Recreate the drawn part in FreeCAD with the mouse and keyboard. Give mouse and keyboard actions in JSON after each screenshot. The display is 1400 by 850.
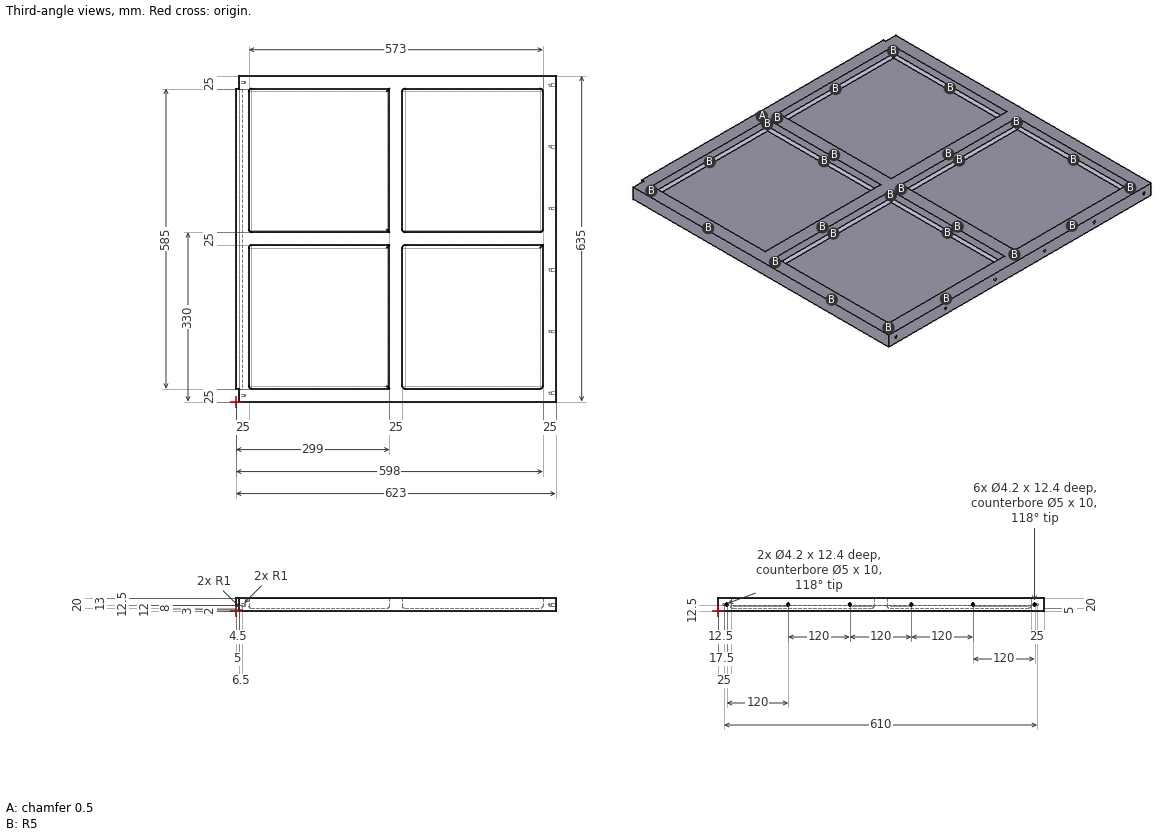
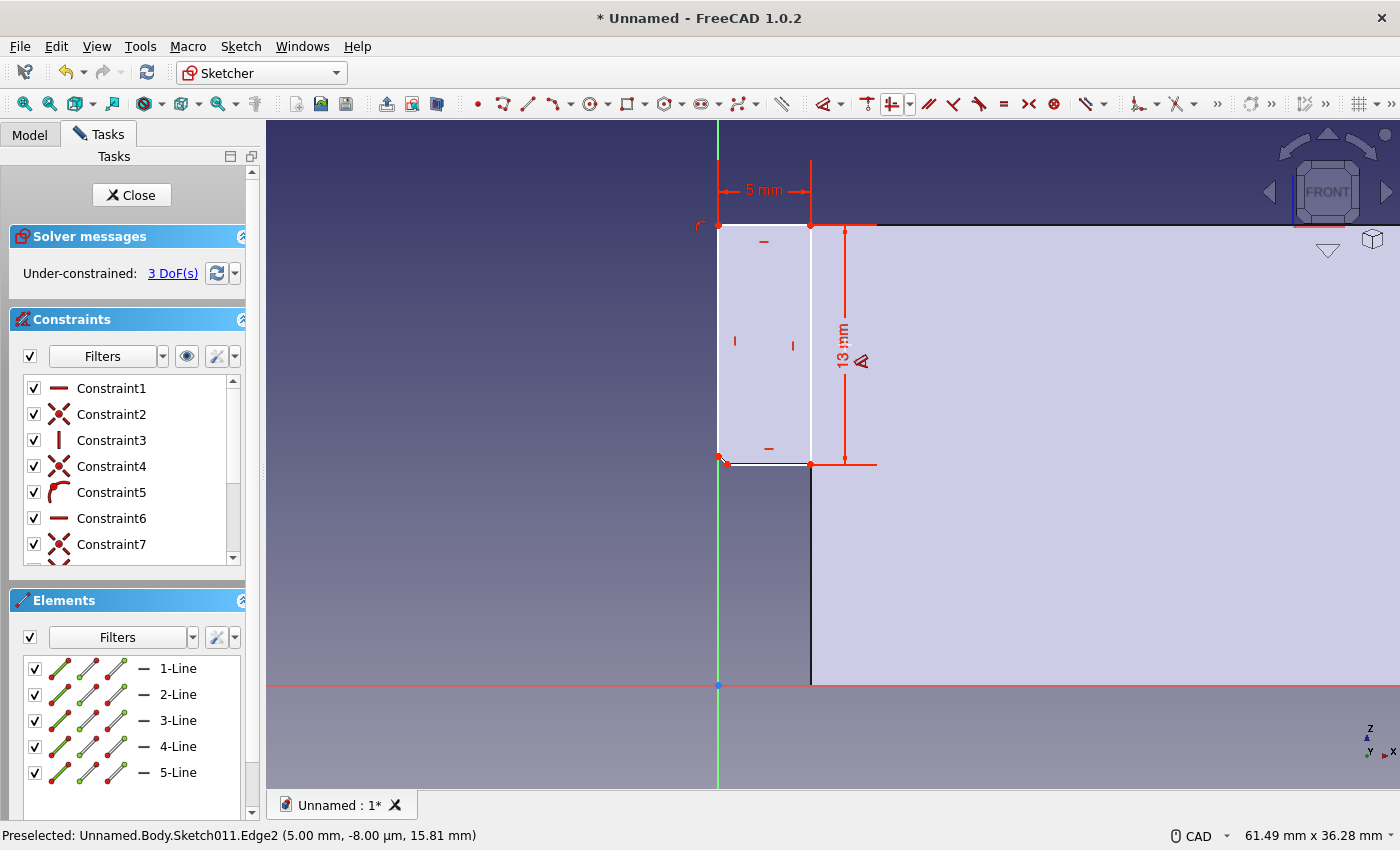
{"action": "left_click", "coordinate": [752, 465]}
{"action": "left_click", "coordinate": [769, 499]}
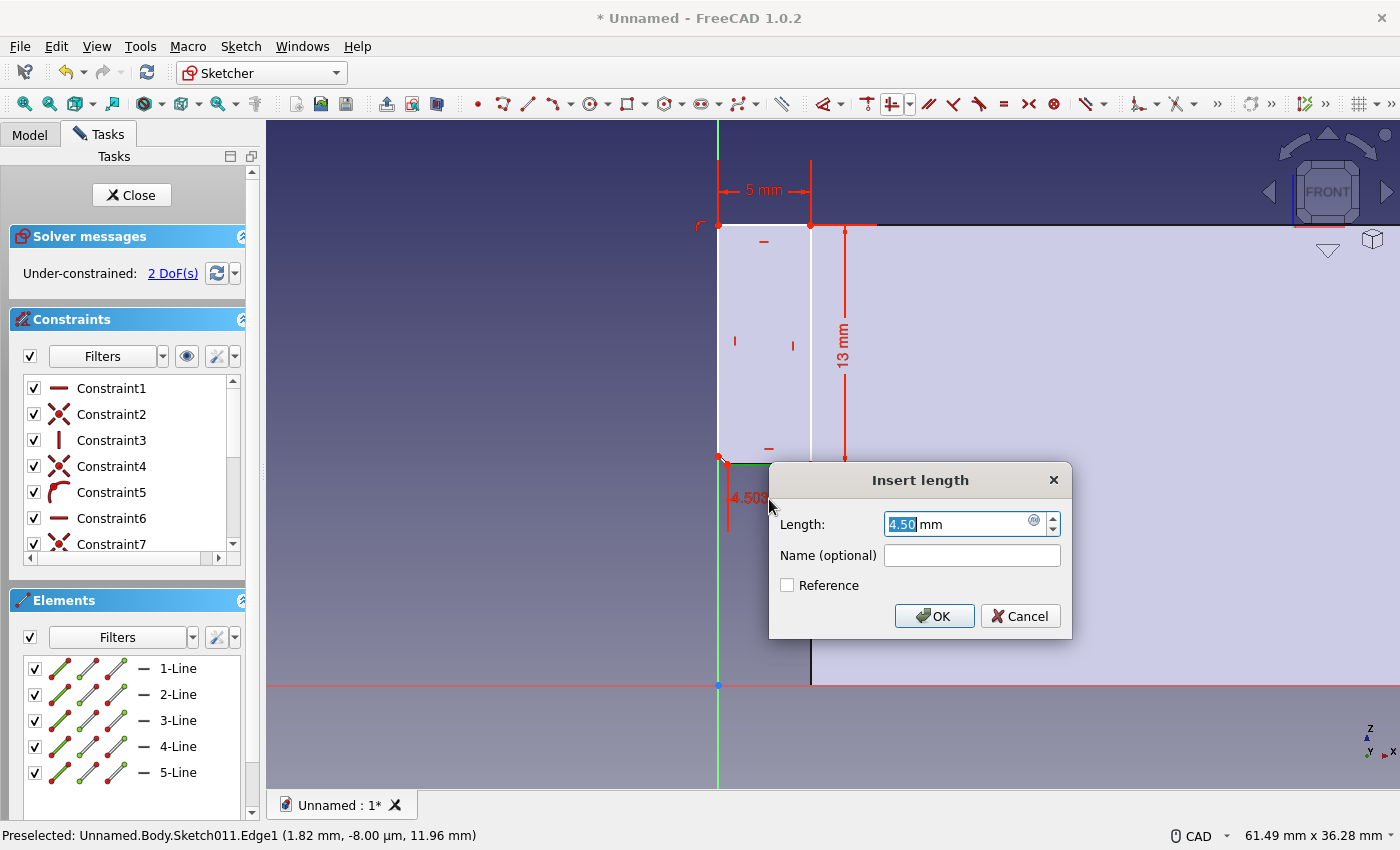
{"action": "type", "text": "4.5"}
{"action": "key", "text": "Return"}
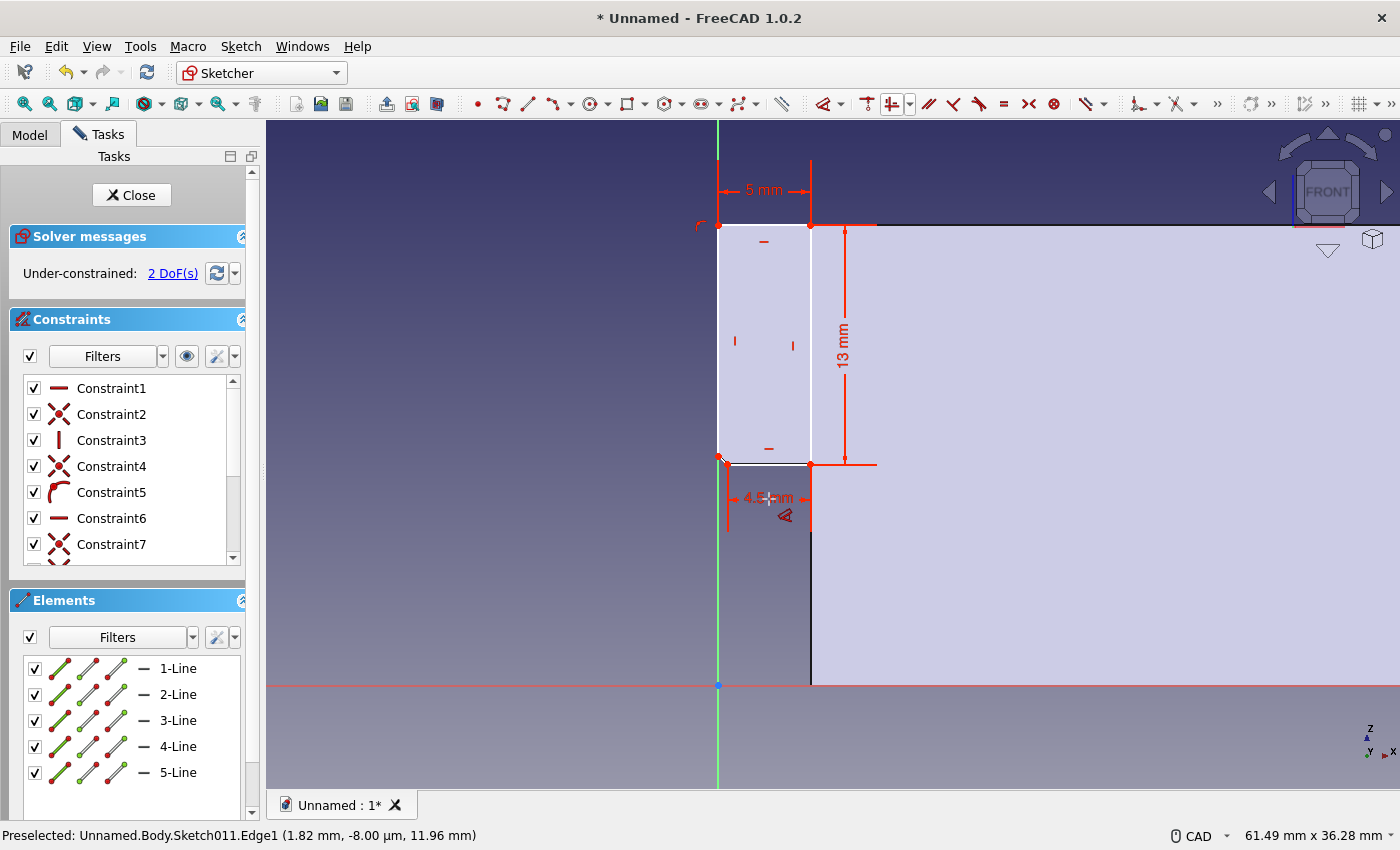
{"action": "left_click", "coordinate": [728, 465]}
{"action": "left_click", "coordinate": [684, 575]}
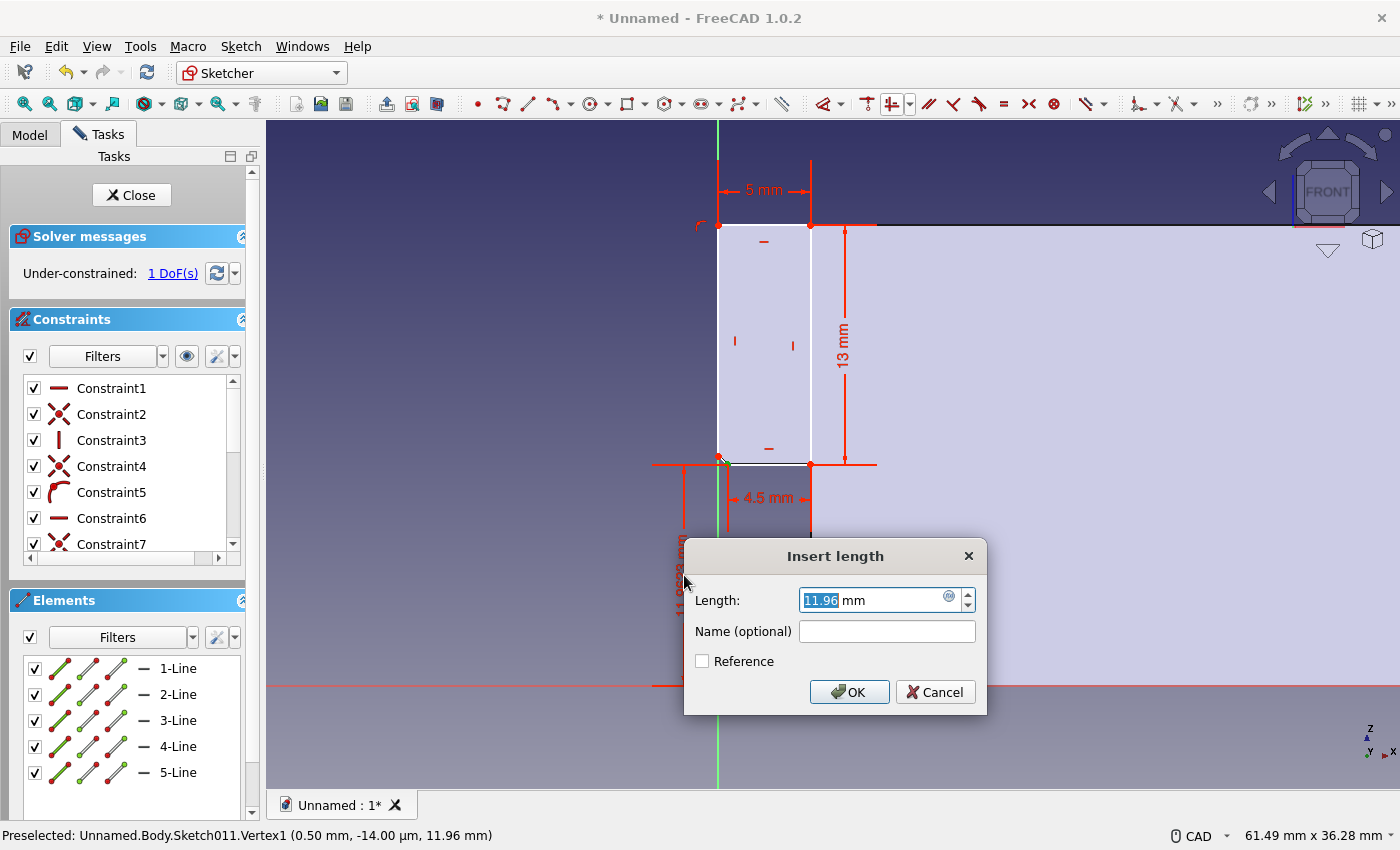
{"action": "type", "text": "12"}
{"action": "key", "text": "Return"}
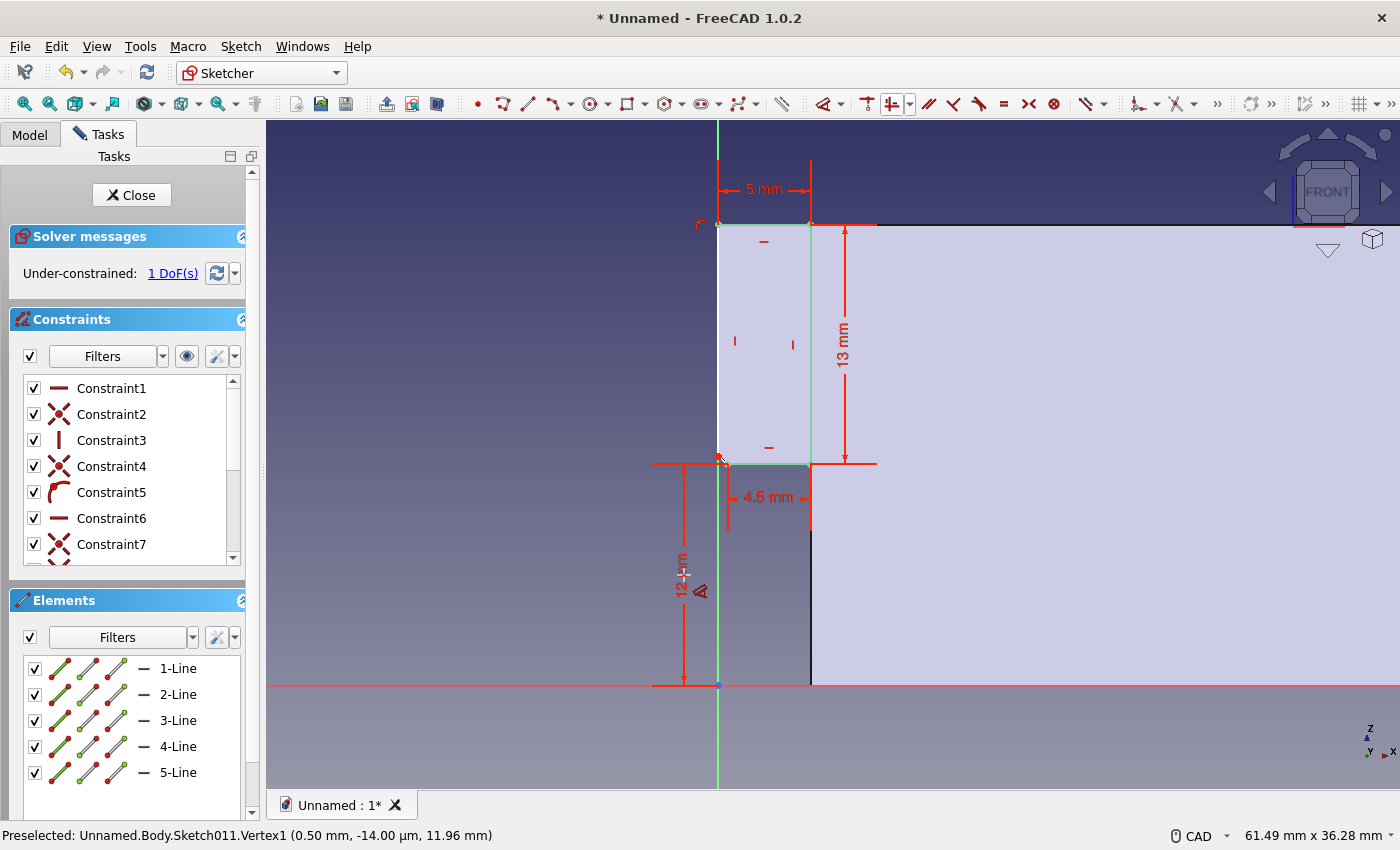
{"action": "left_click", "coordinate": [718, 294]}
{"action": "left_click", "coordinate": [684, 340]}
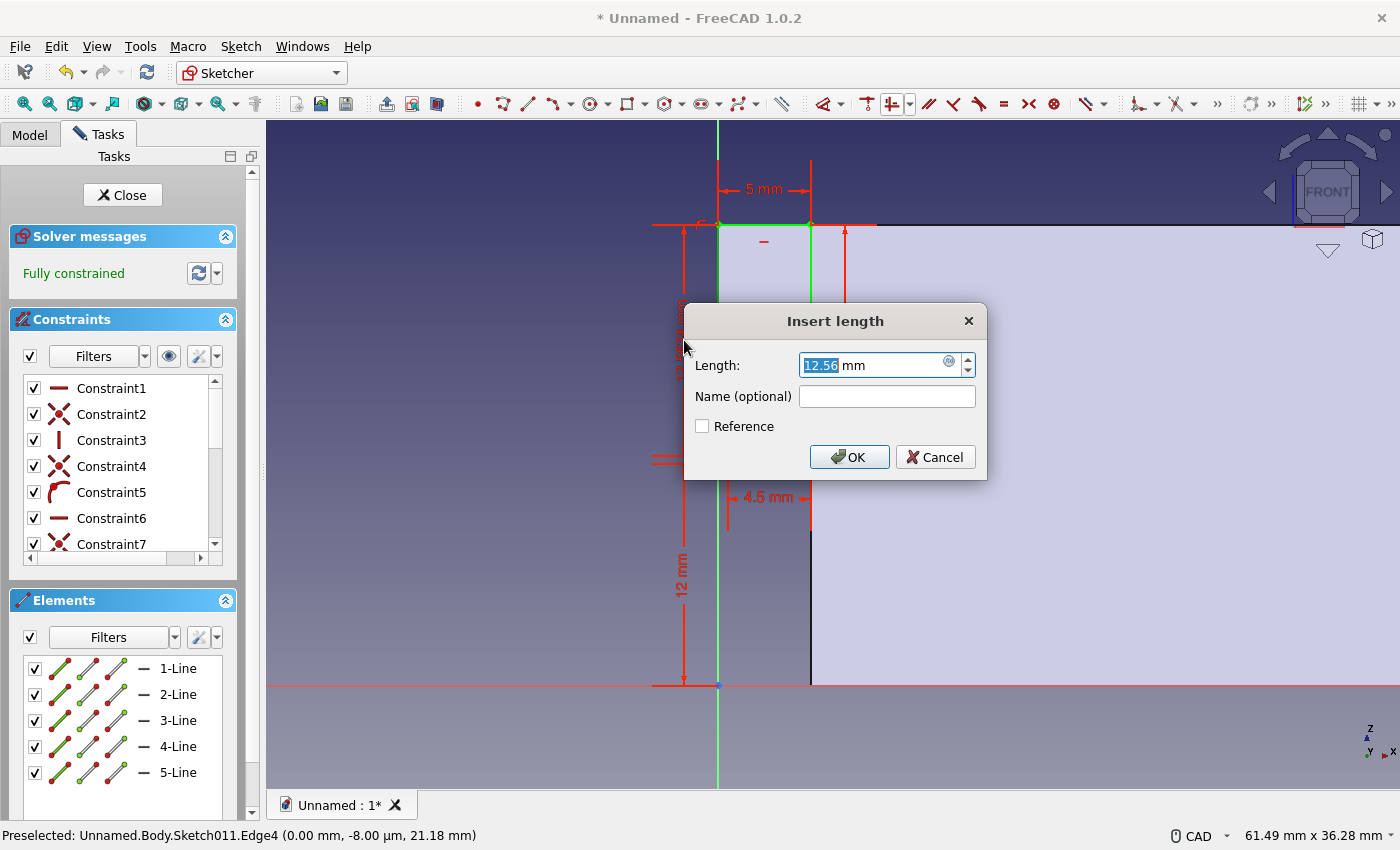
{"action": "type", "text": "12.5"}
{"action": "key", "text": "Return"}
{"action": "key", "text": "Escape"}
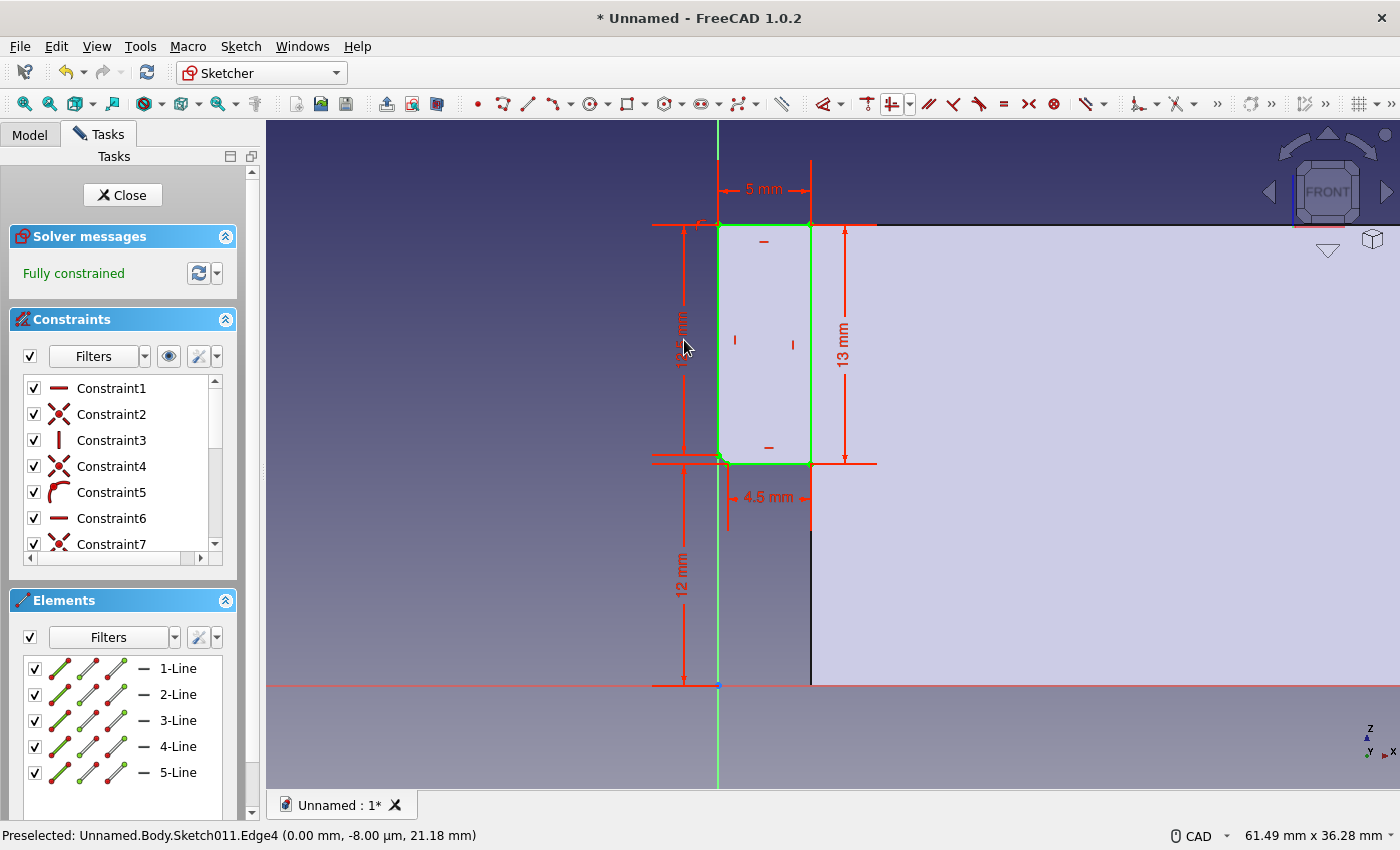
{"action": "left_click", "coordinate": [123, 195]}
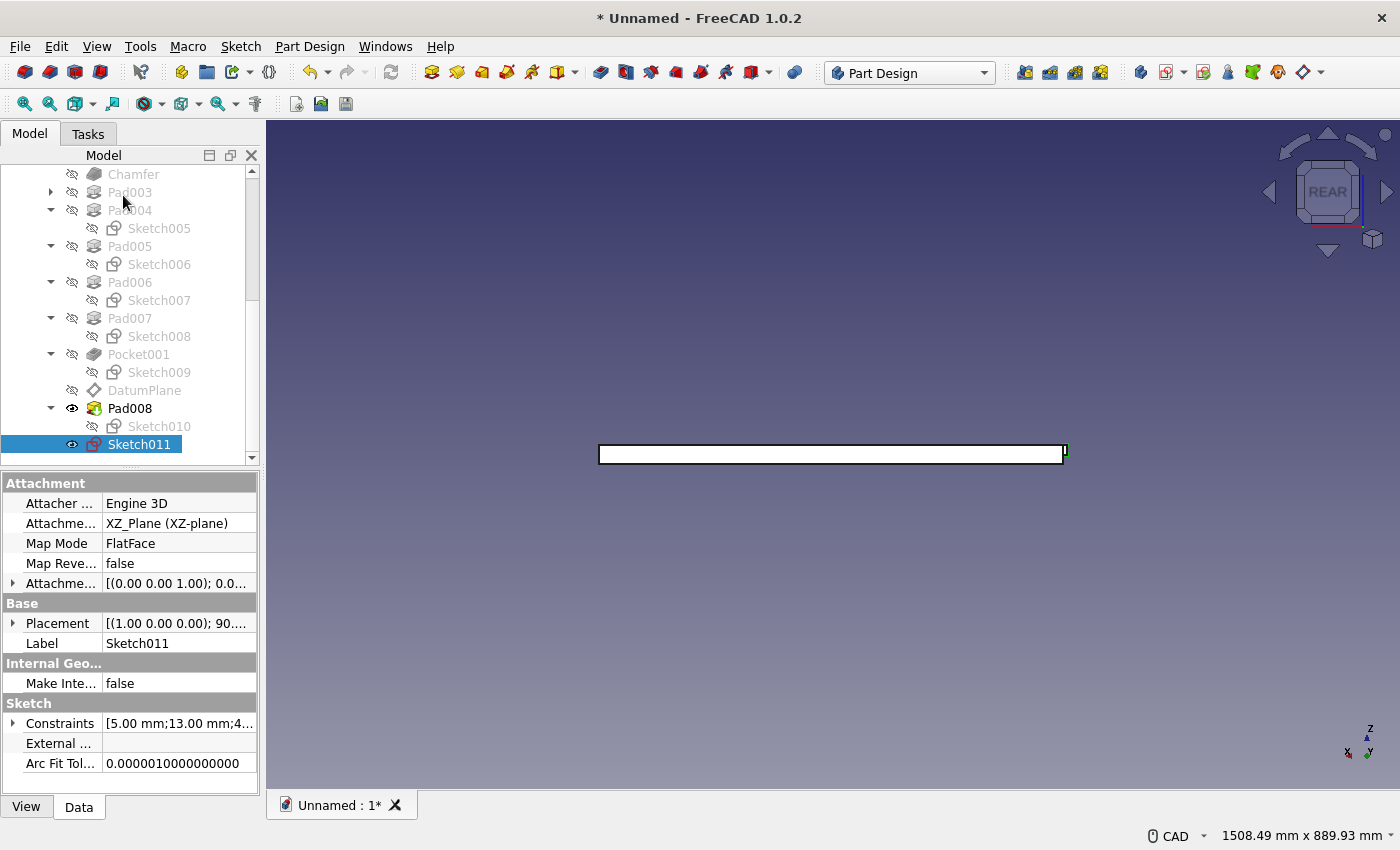
{"action": "left_click", "coordinate": [601, 72]}